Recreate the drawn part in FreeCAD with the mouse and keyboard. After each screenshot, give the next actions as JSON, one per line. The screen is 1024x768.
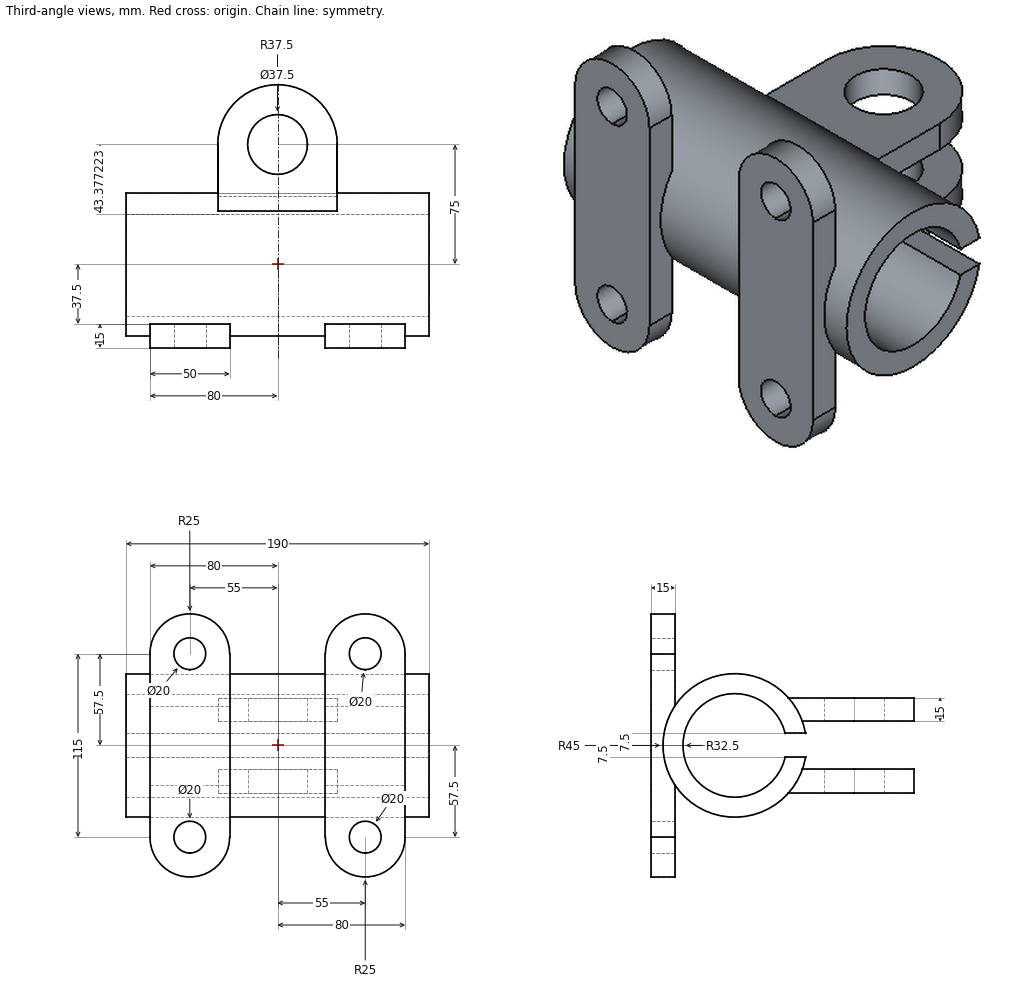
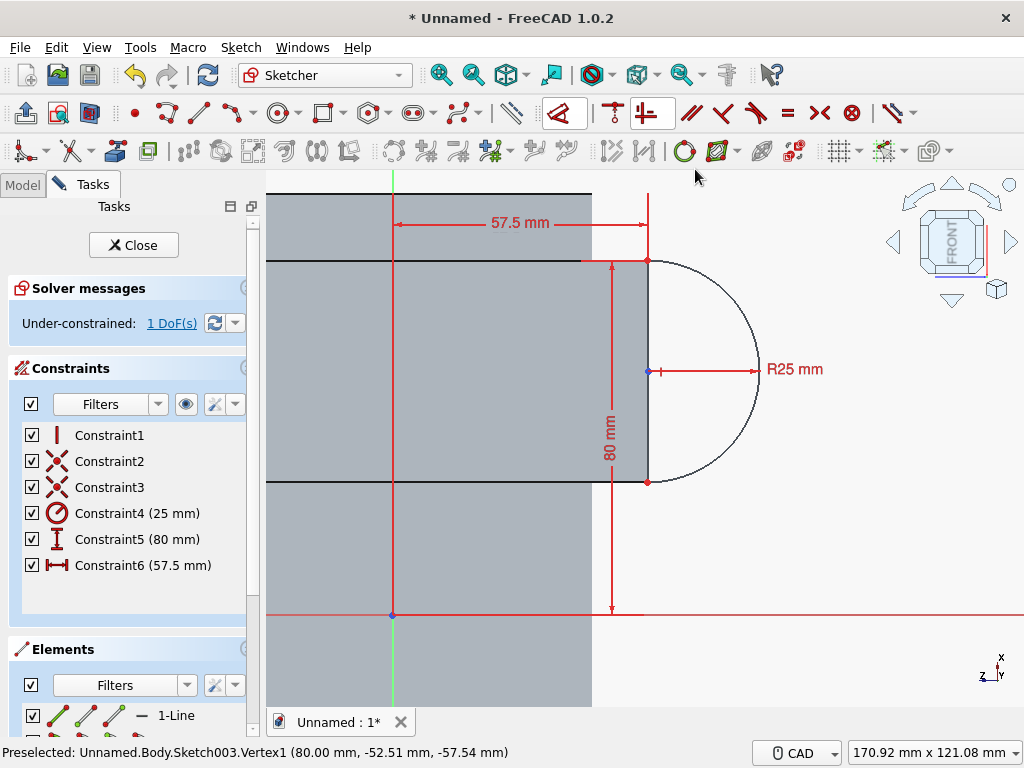
{"action": "left_click", "coordinate": [649, 371]}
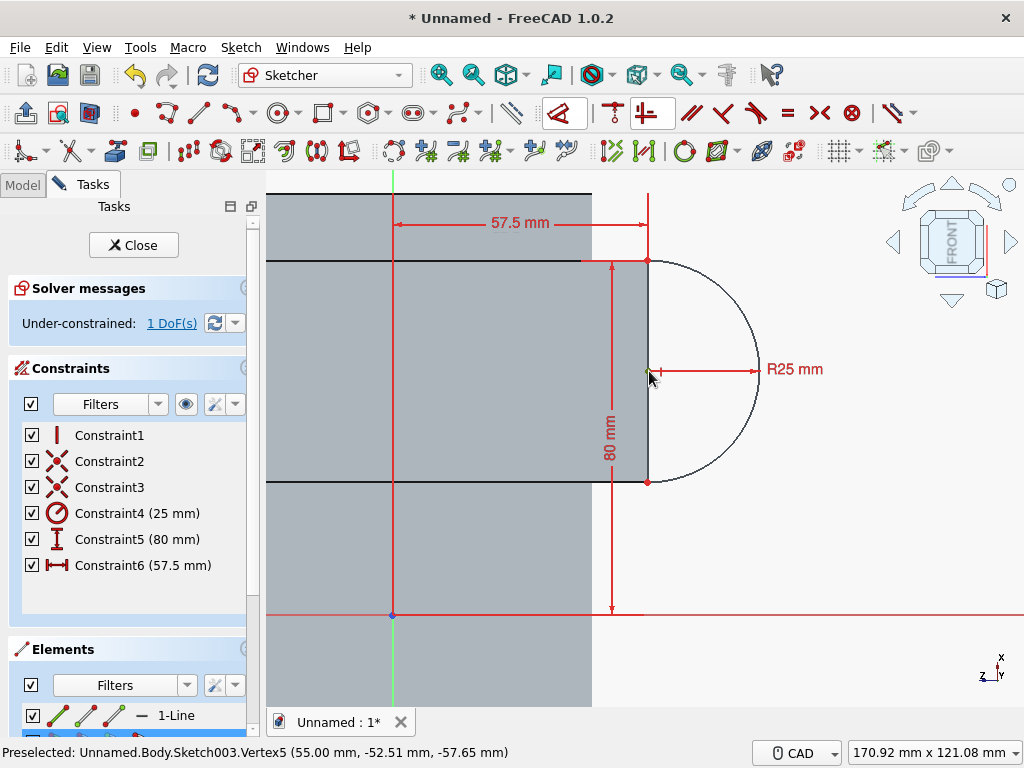
{"action": "left_click", "coordinate": [582, 114]}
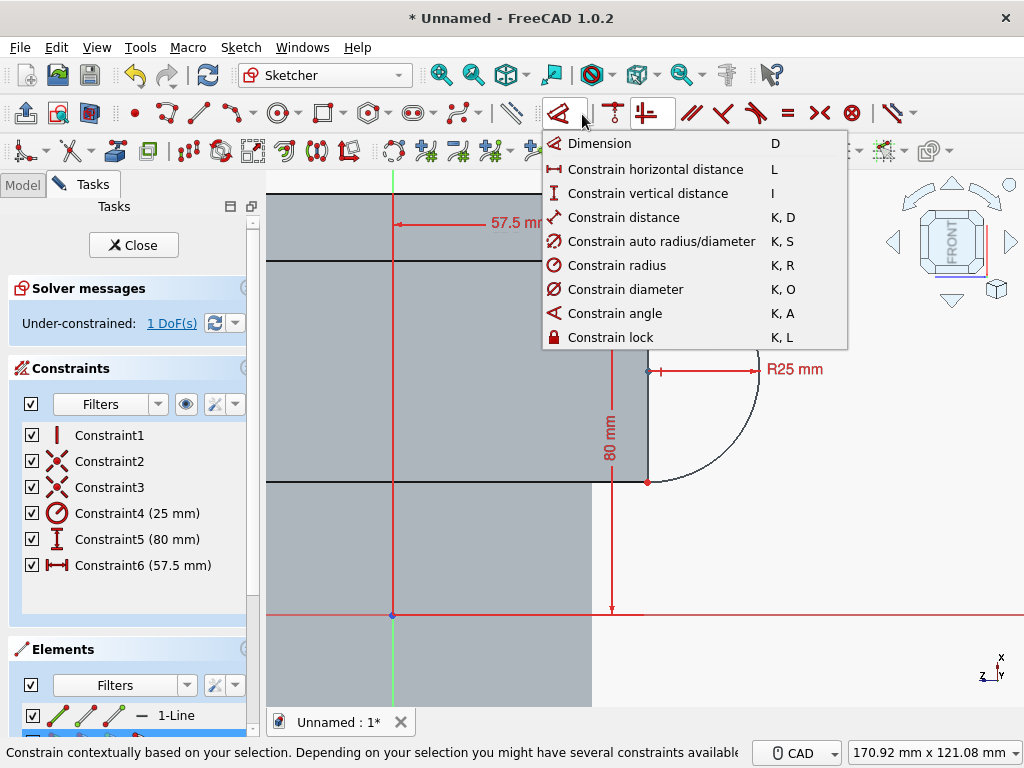
{"action": "left_click", "coordinate": [695, 169]}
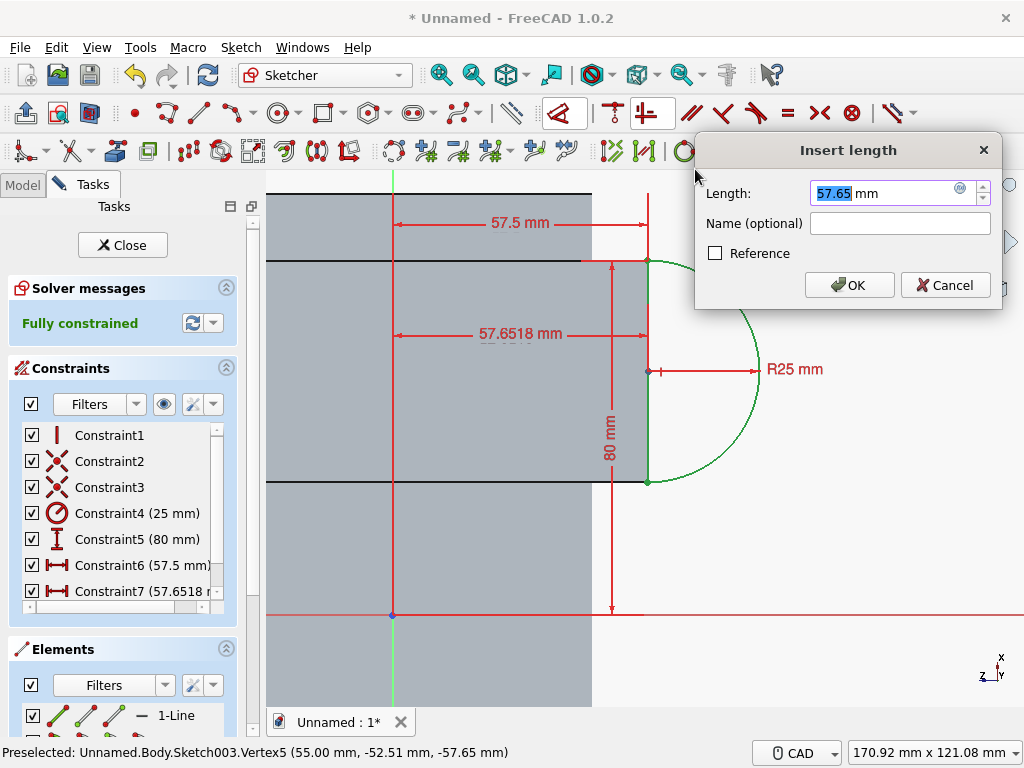
{"action": "type", "text": "57.5"}
{"action": "key", "text": "Return"}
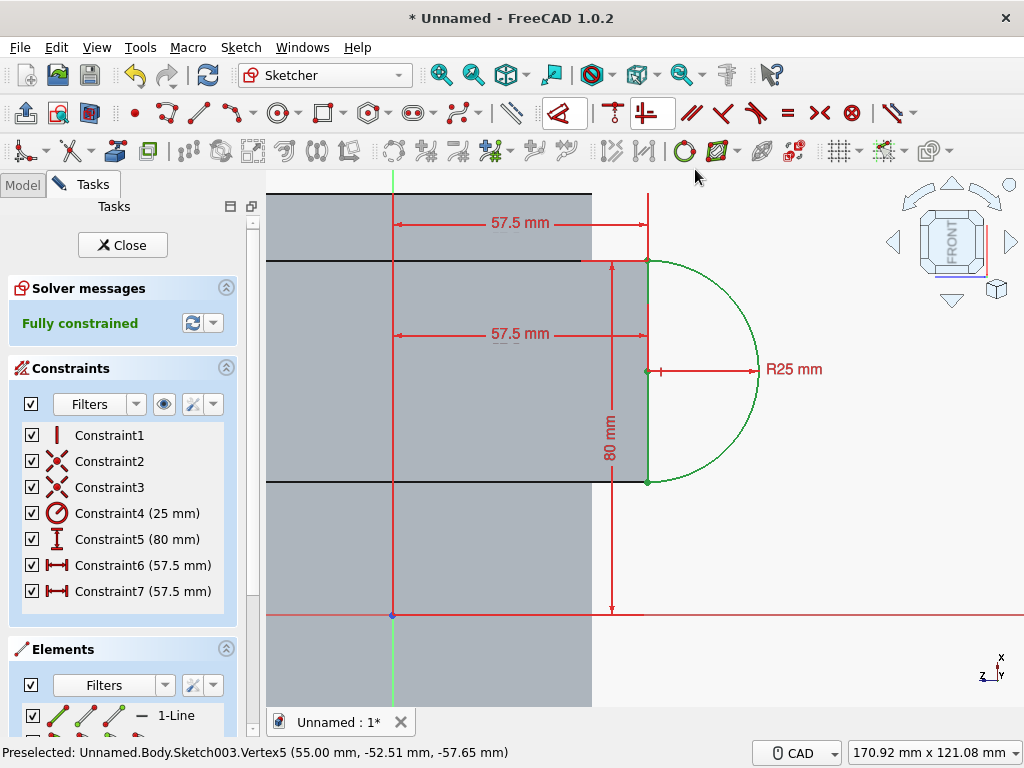
{"action": "left_click", "coordinate": [123, 245]}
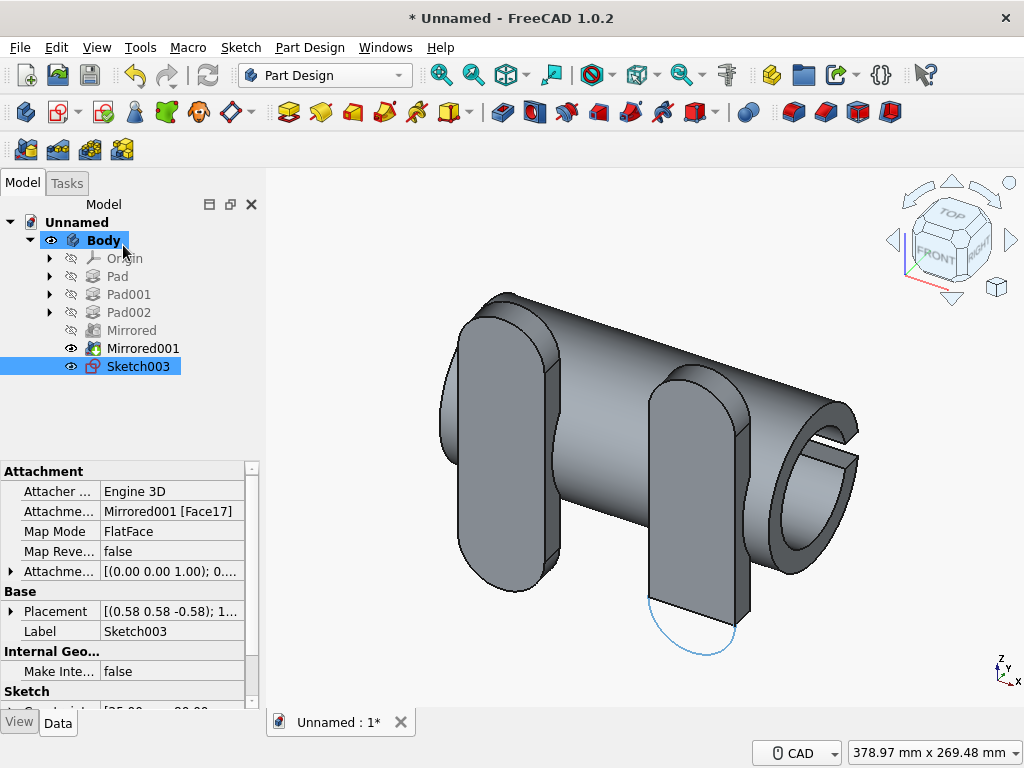
{"action": "left_click", "coordinate": [290, 112]}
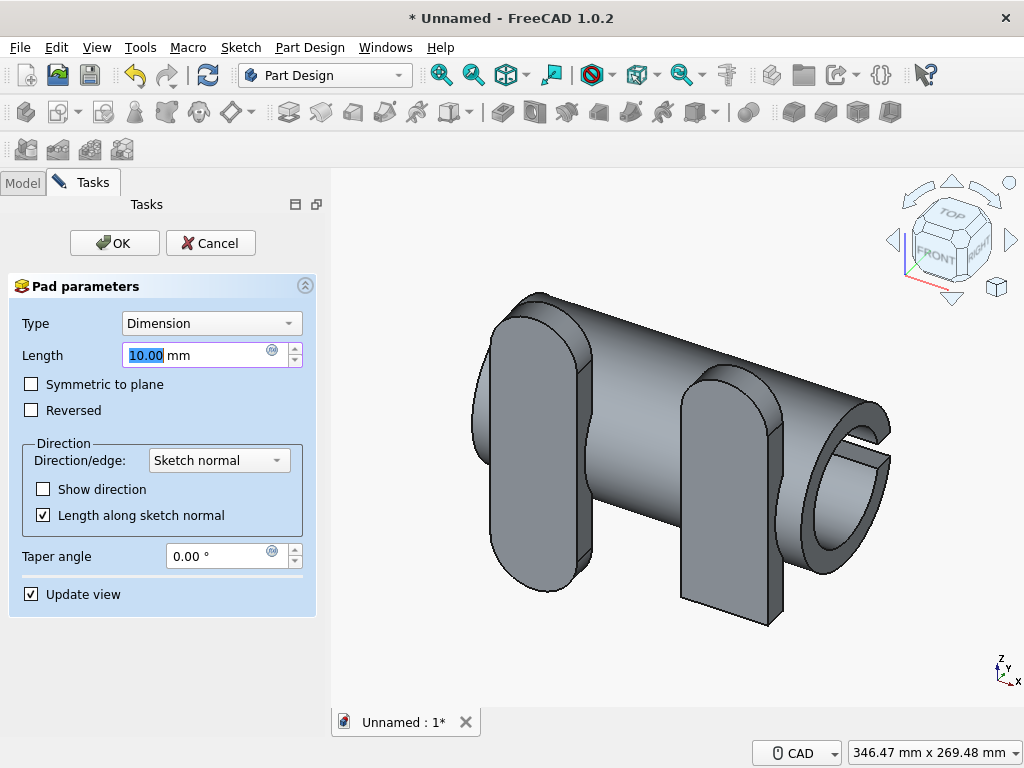
{"action": "type", "text": "15"}
{"action": "key", "text": "Tab"}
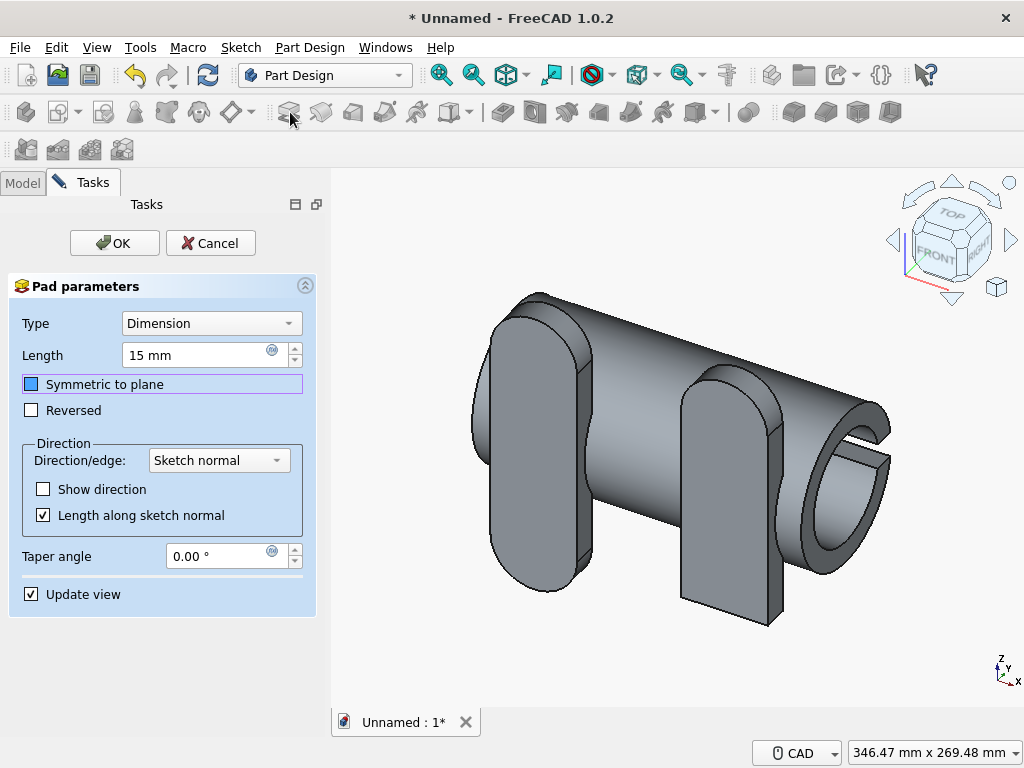
{"action": "left_click", "coordinate": [30, 410]}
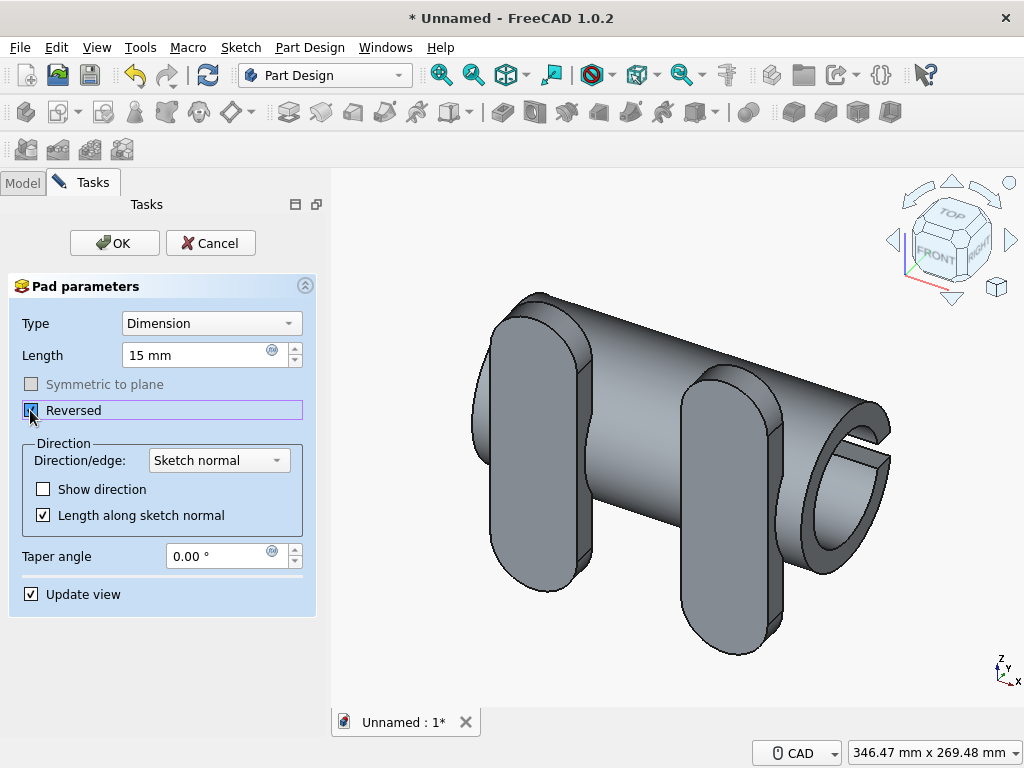
{"action": "left_click", "coordinate": [115, 243]}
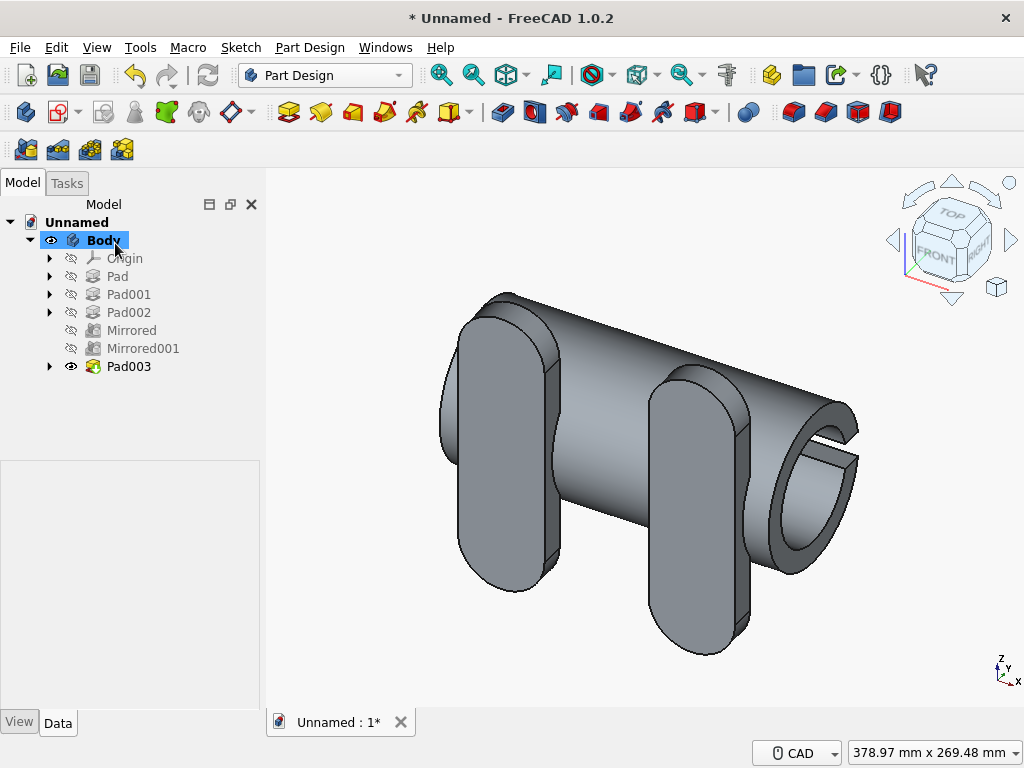
{"action": "left_click", "coordinate": [692, 516]}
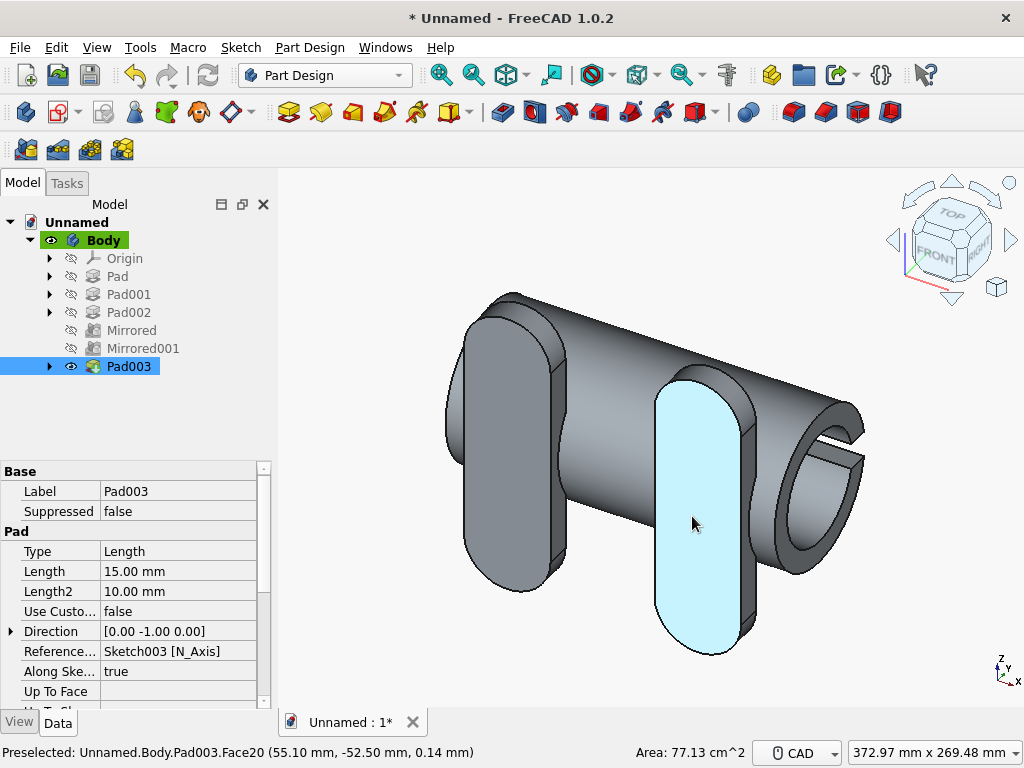
{"action": "left_click", "coordinate": [58, 112]}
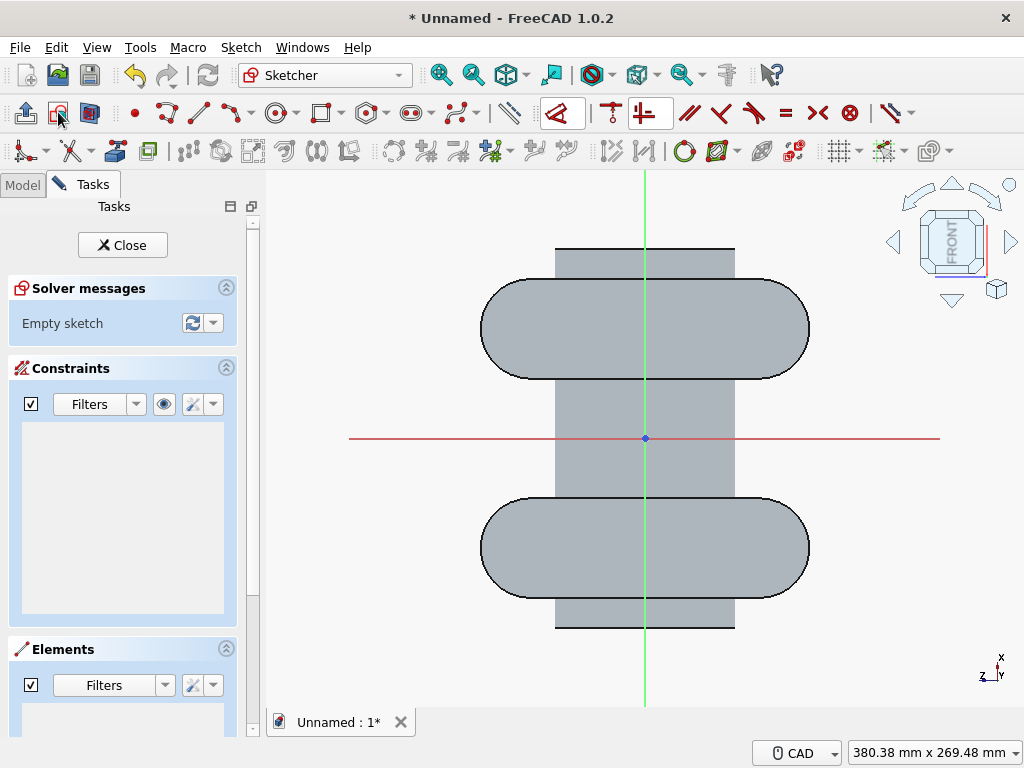
{"action": "scroll", "coordinate": [525, 562], "scroll_direction": "up", "scroll_amount": 11}